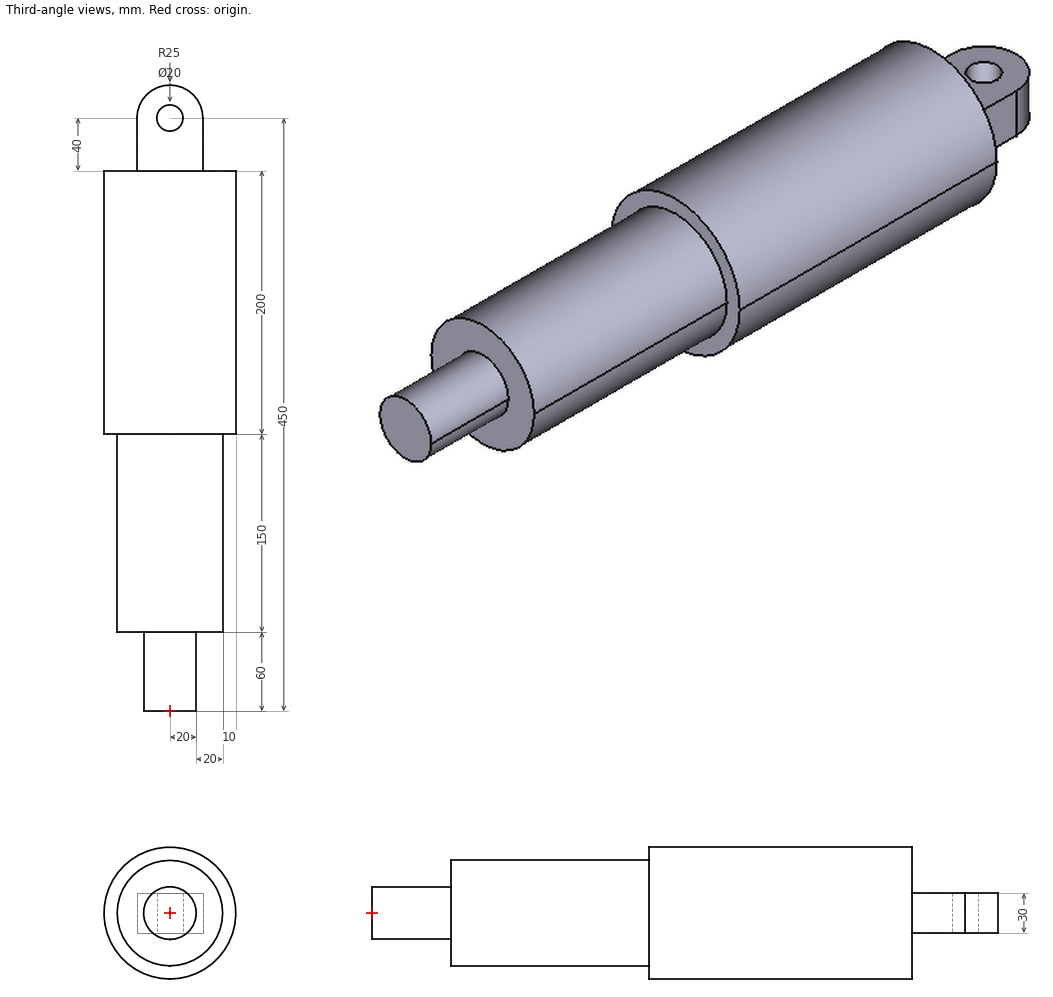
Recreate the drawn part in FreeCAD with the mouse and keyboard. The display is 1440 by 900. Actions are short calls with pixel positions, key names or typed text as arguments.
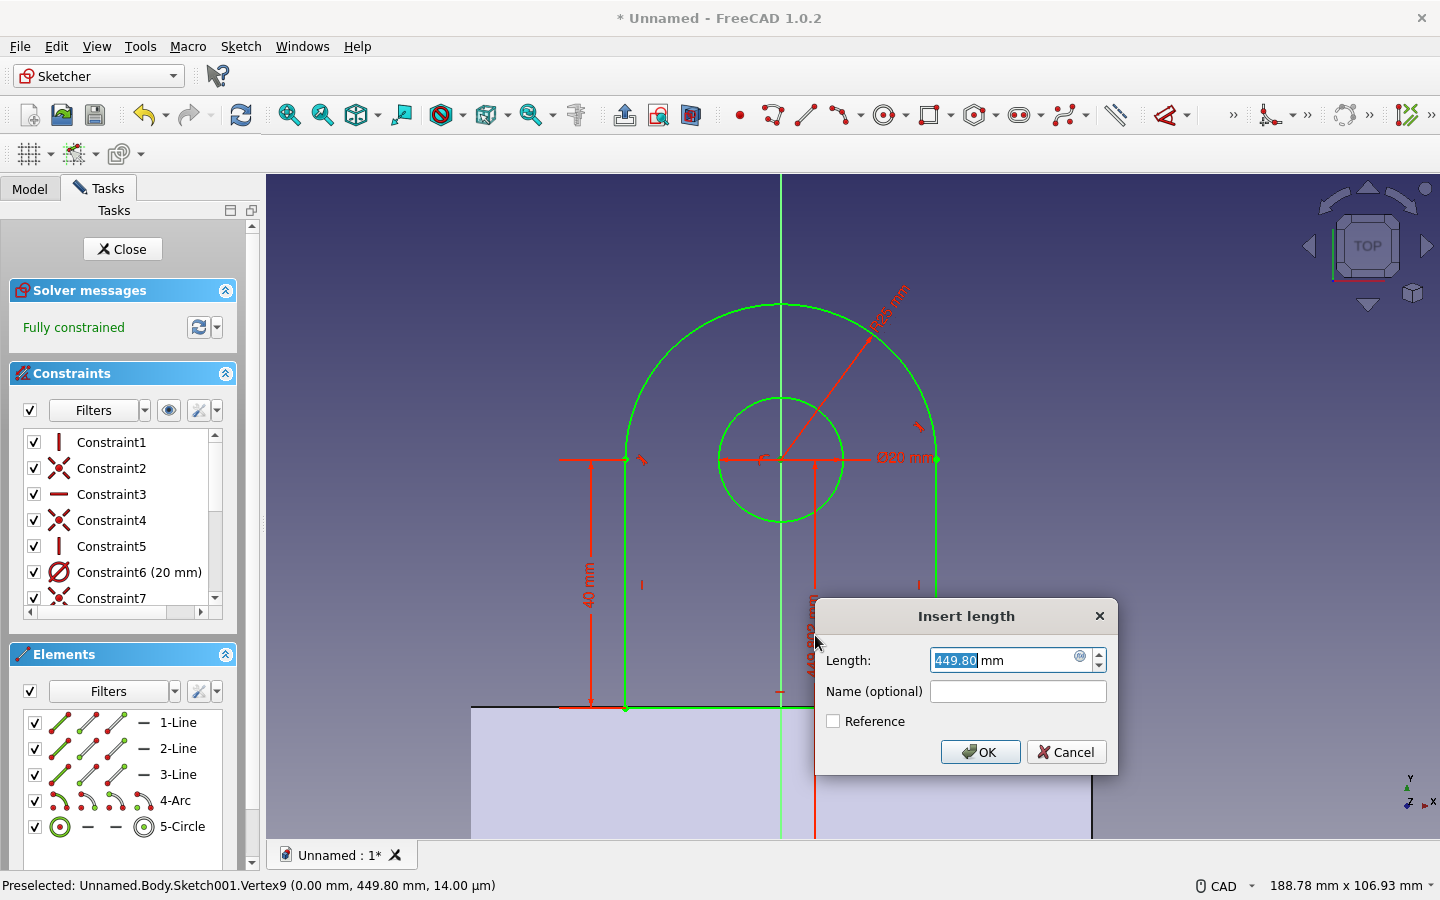
text(450)
key(Return)
key(Escape)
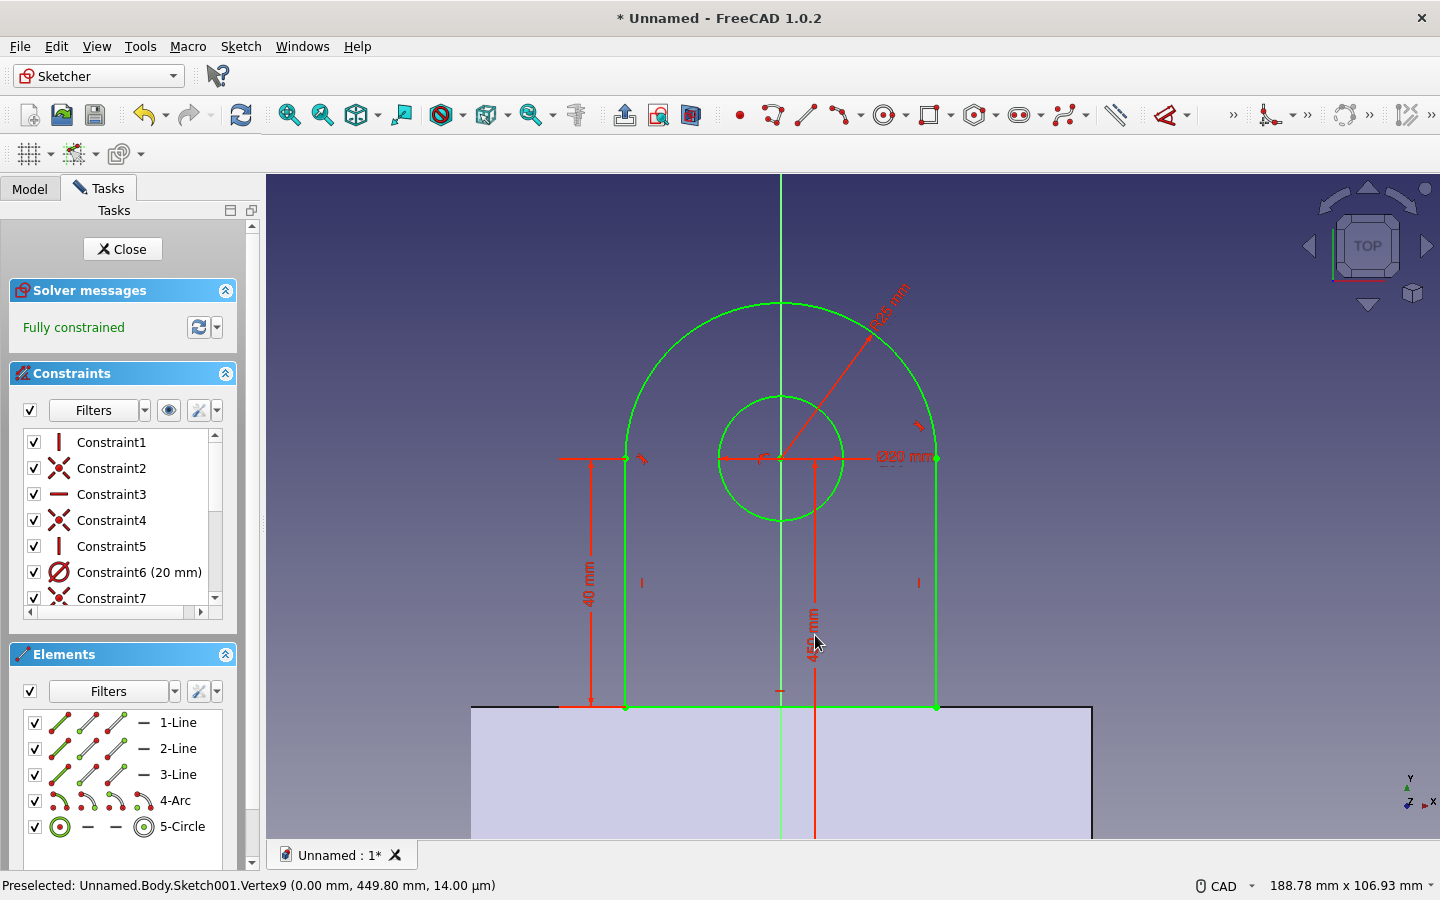
click(123, 249)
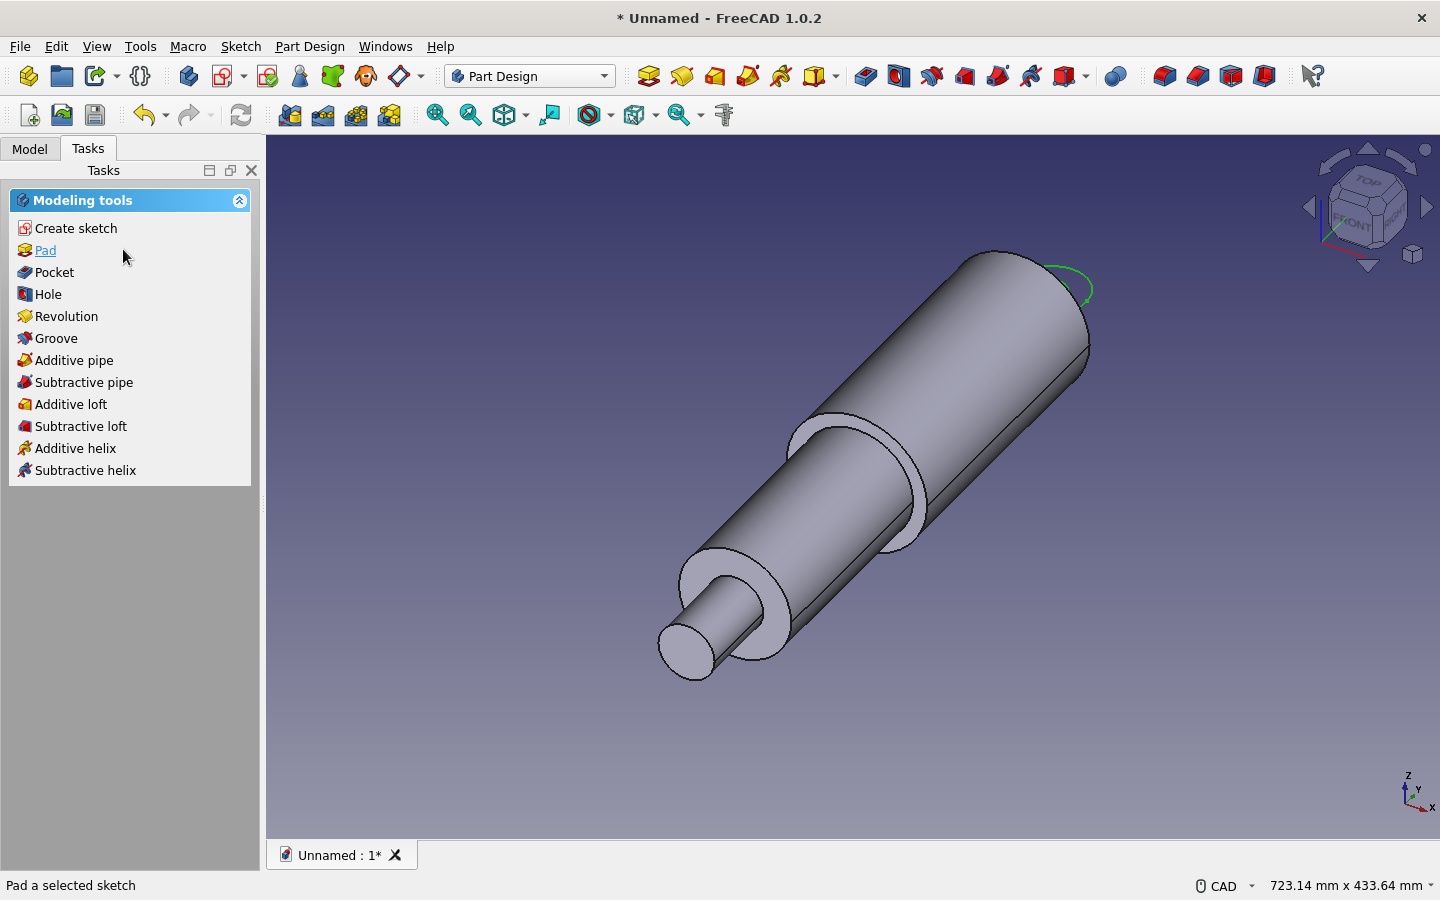
click(649, 76)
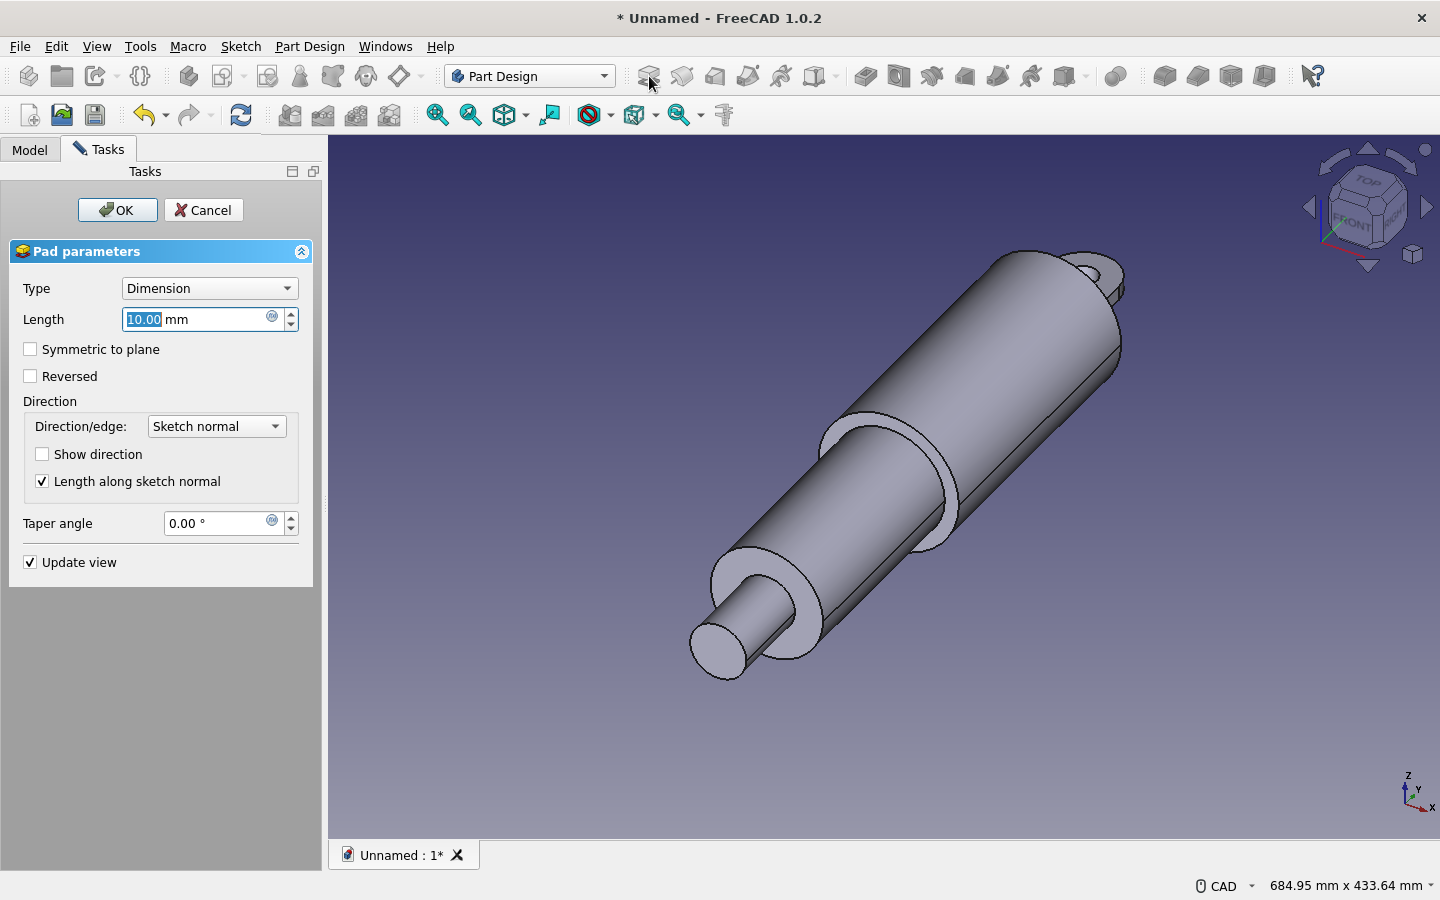
text(30)
key(Tab)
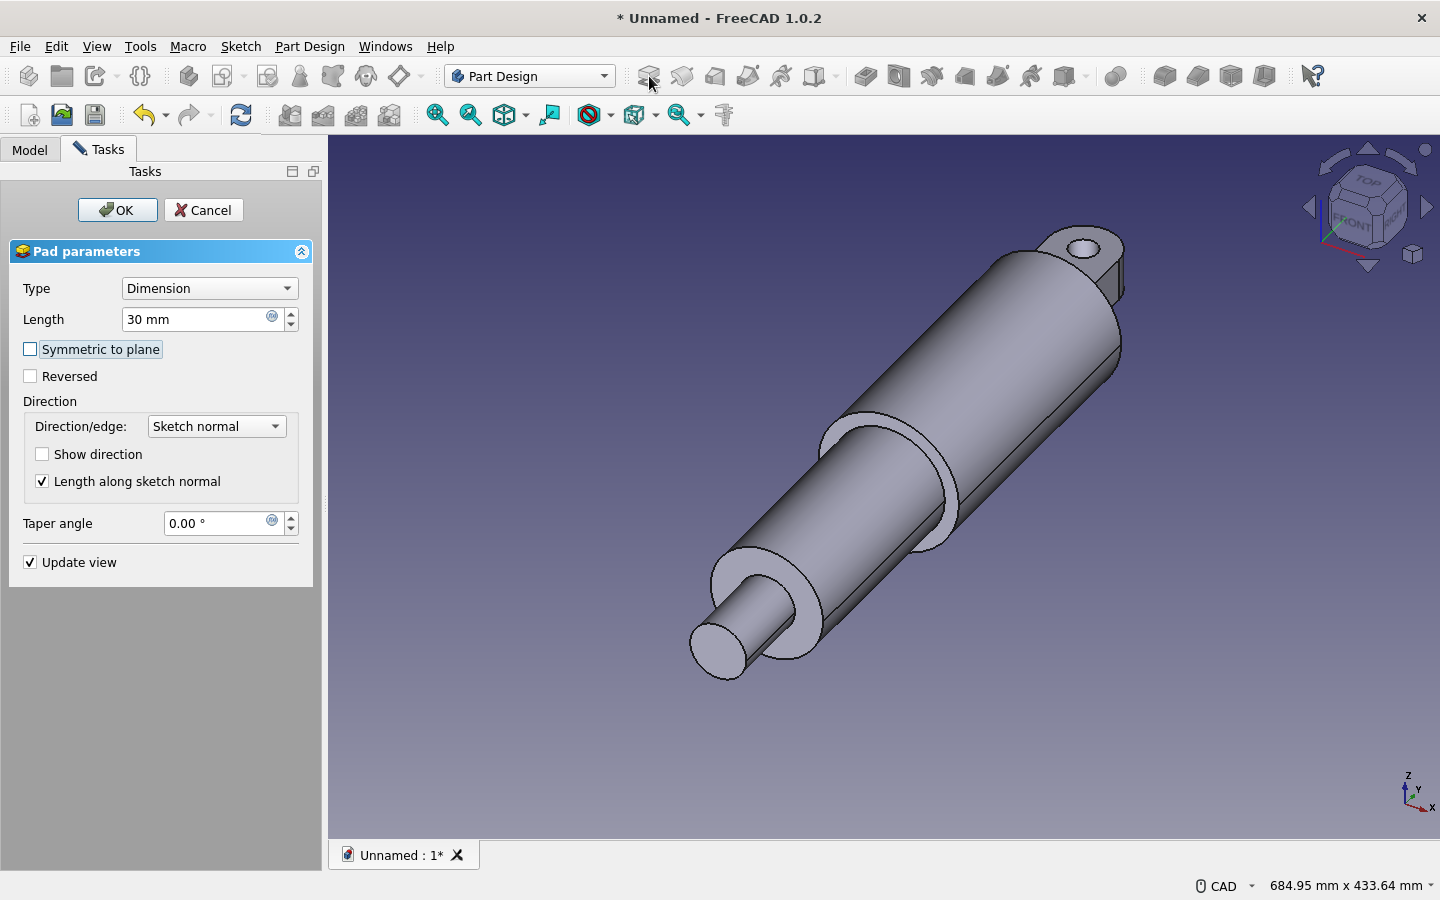
click(31, 349)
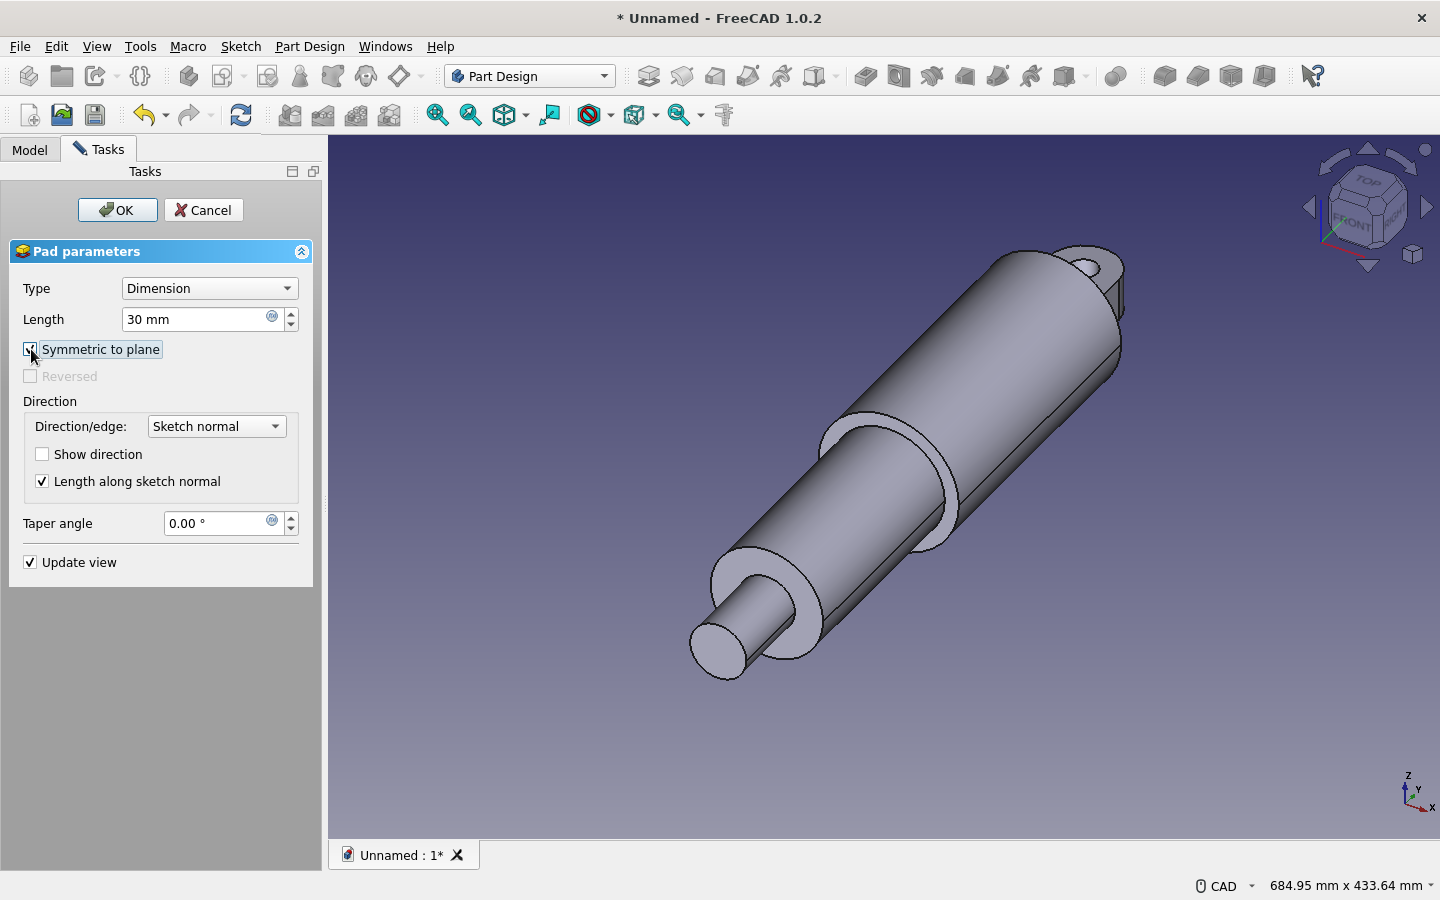
click(118, 210)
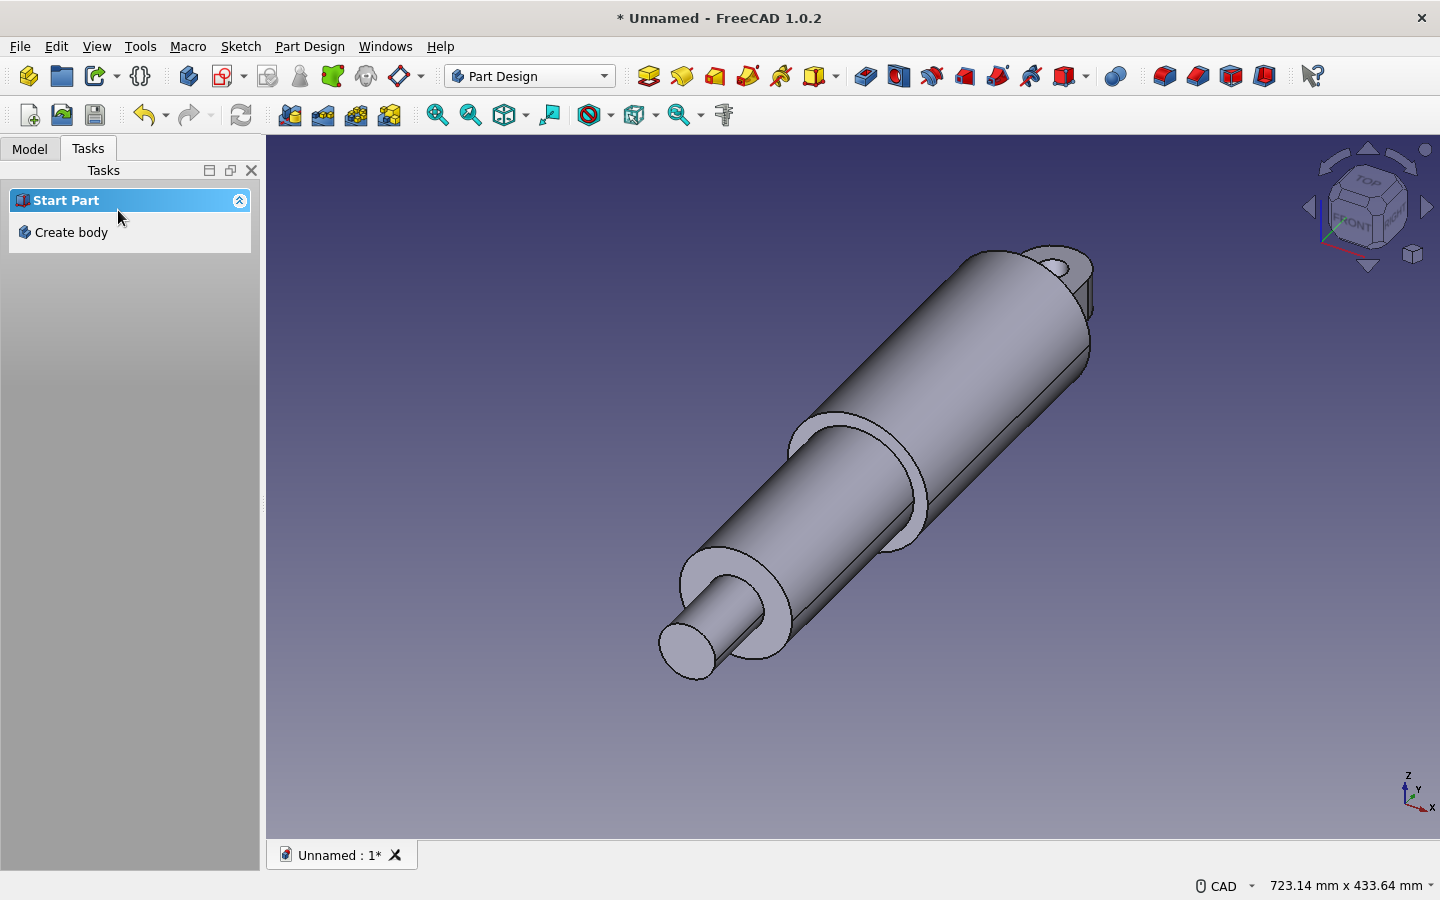
key(0)